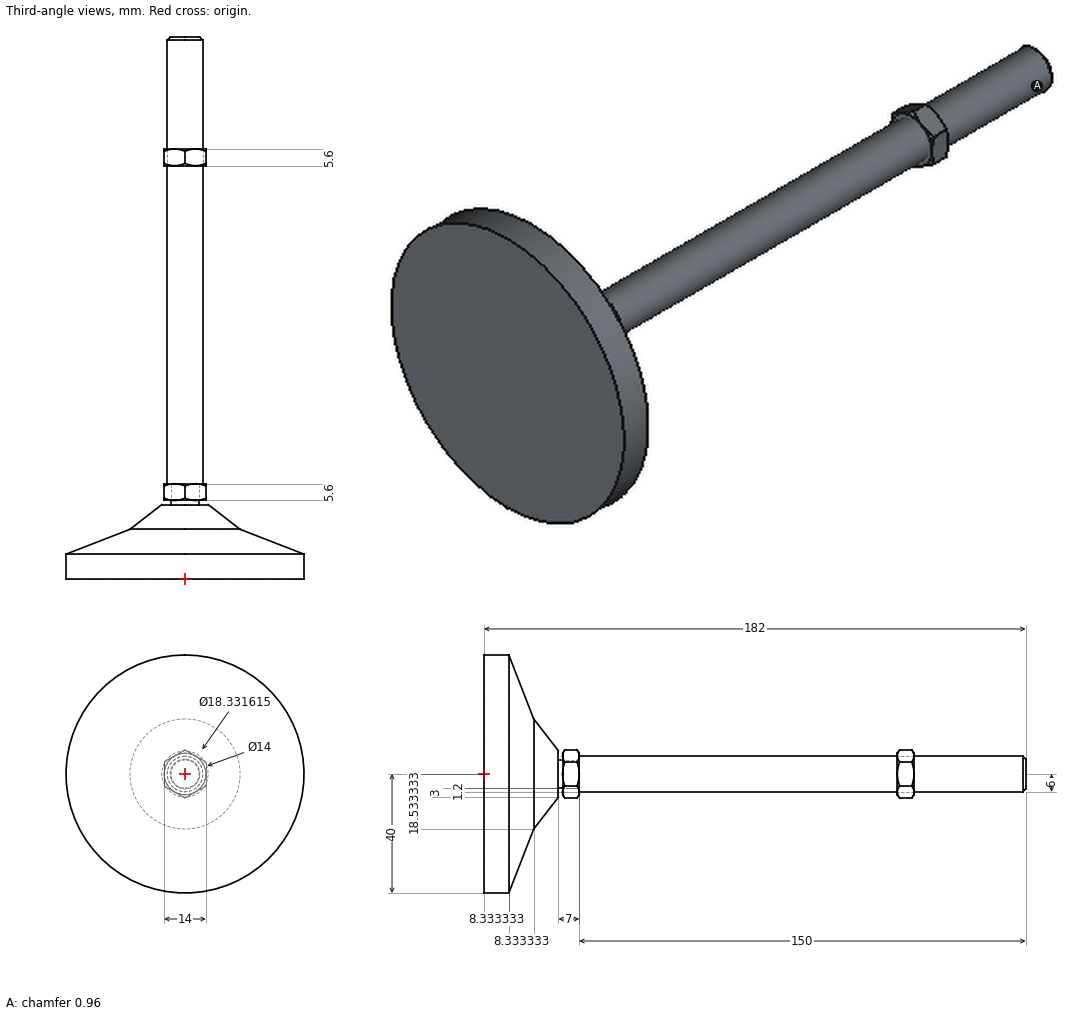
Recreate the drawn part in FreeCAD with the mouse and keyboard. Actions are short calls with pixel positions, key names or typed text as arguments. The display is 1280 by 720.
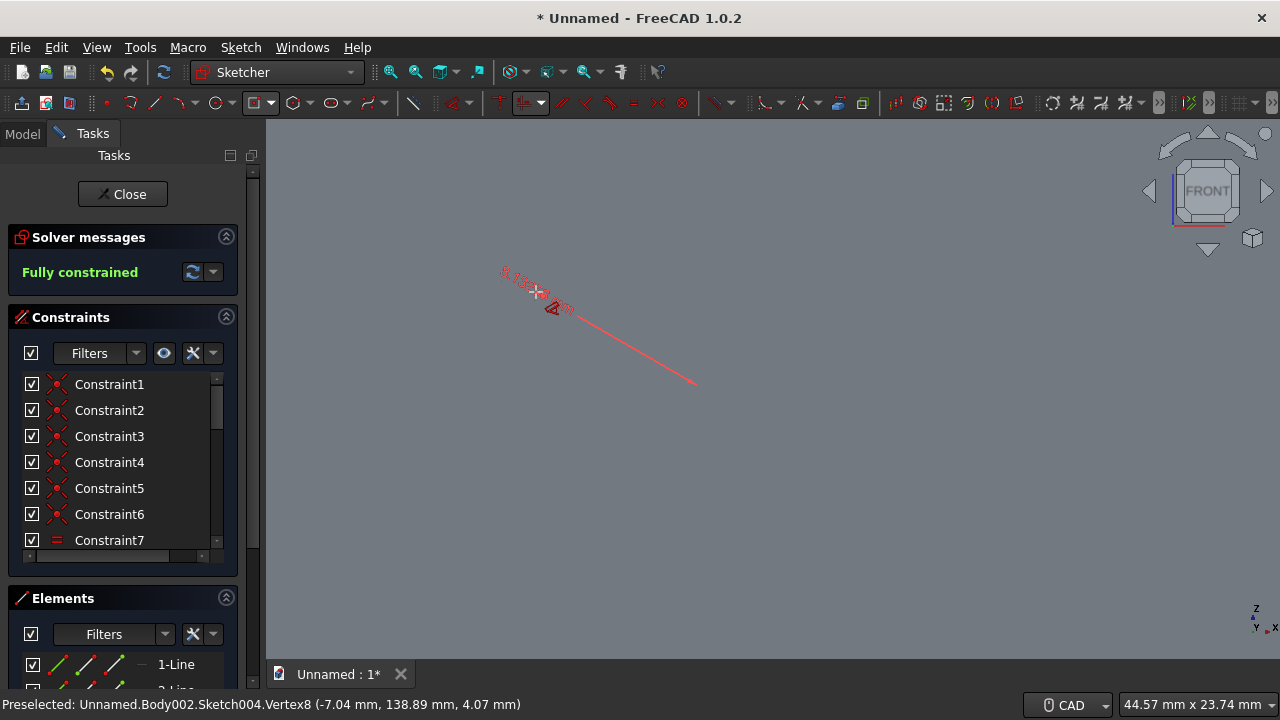
click(857, 477)
click(623, 511)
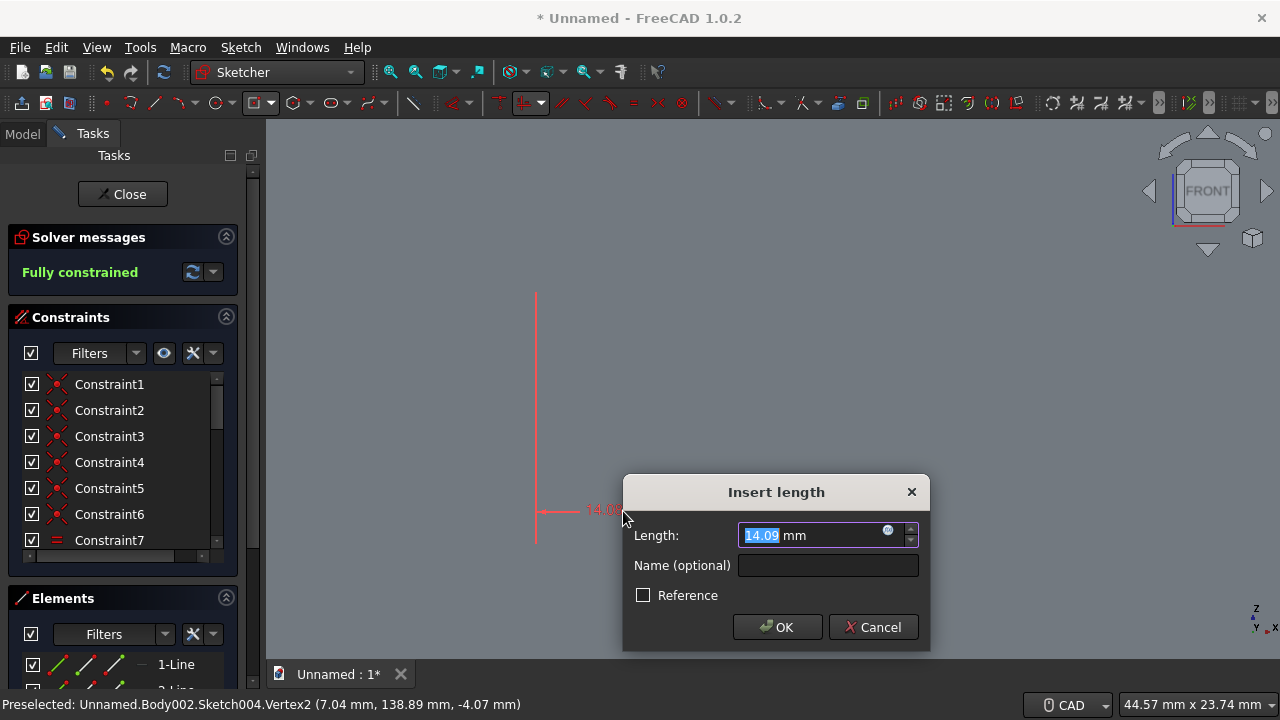
text(14)
key(Return)
key(Escape)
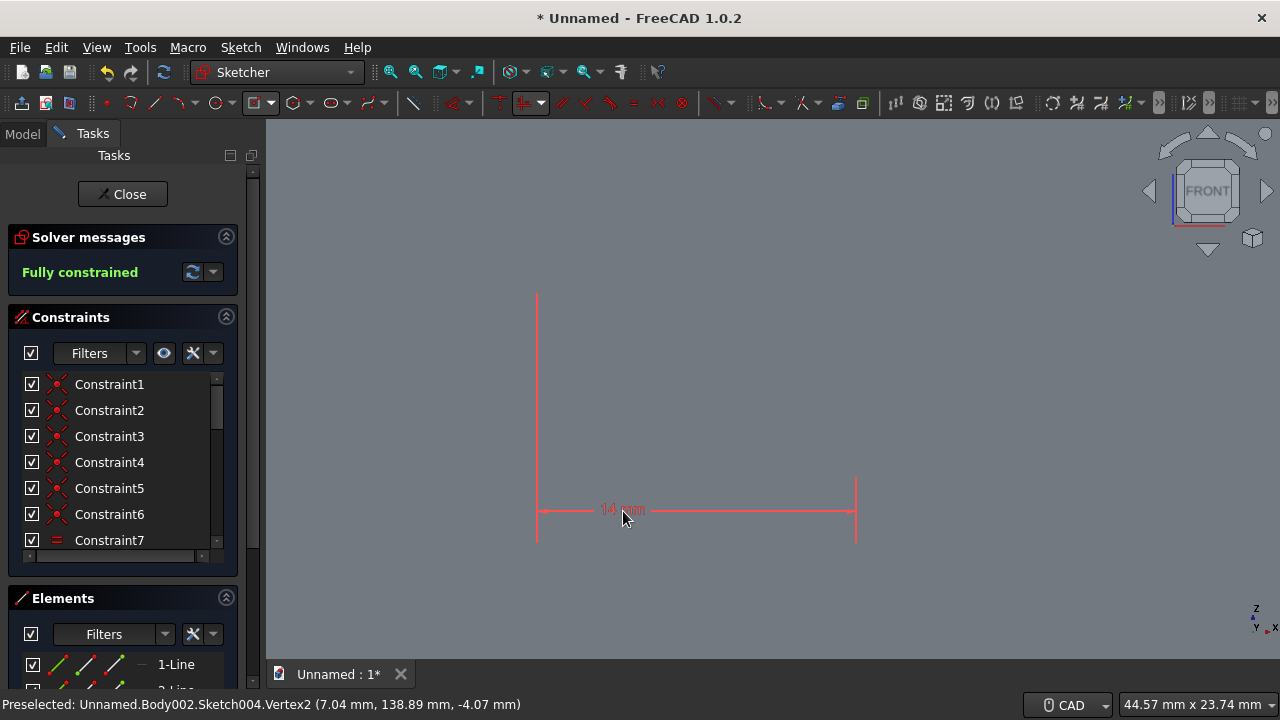
click(123, 194)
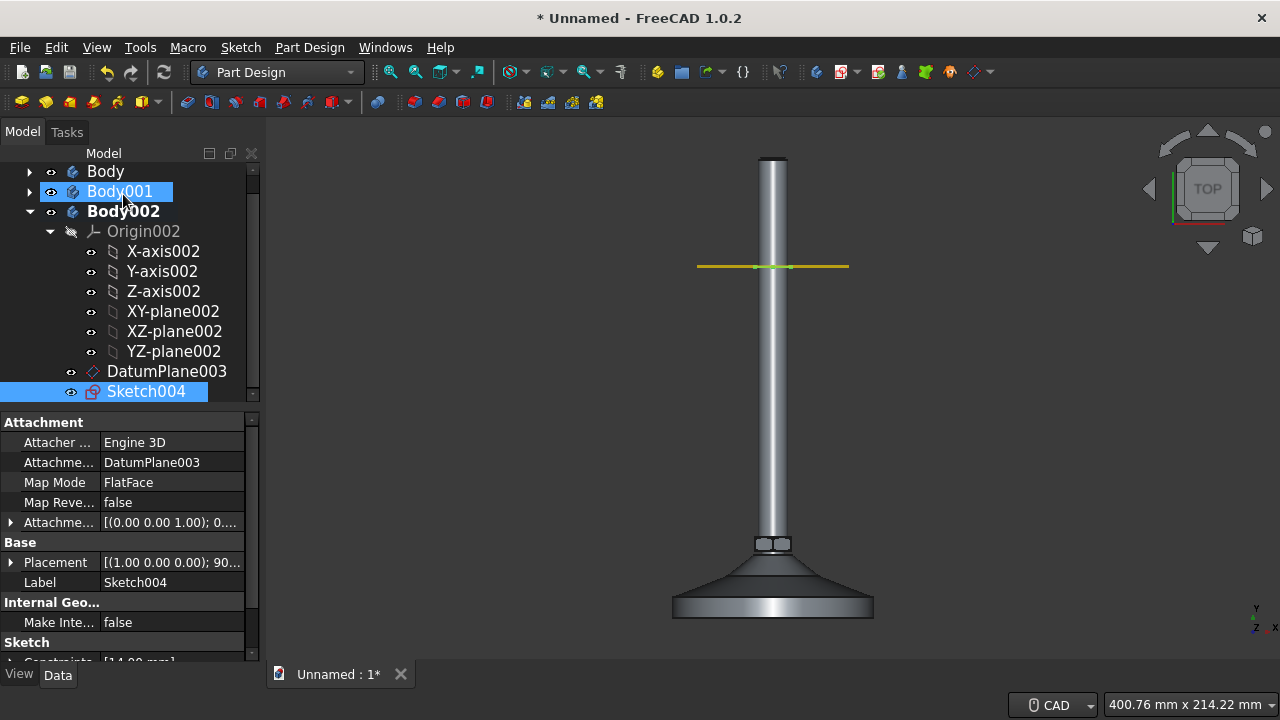
click(22, 102)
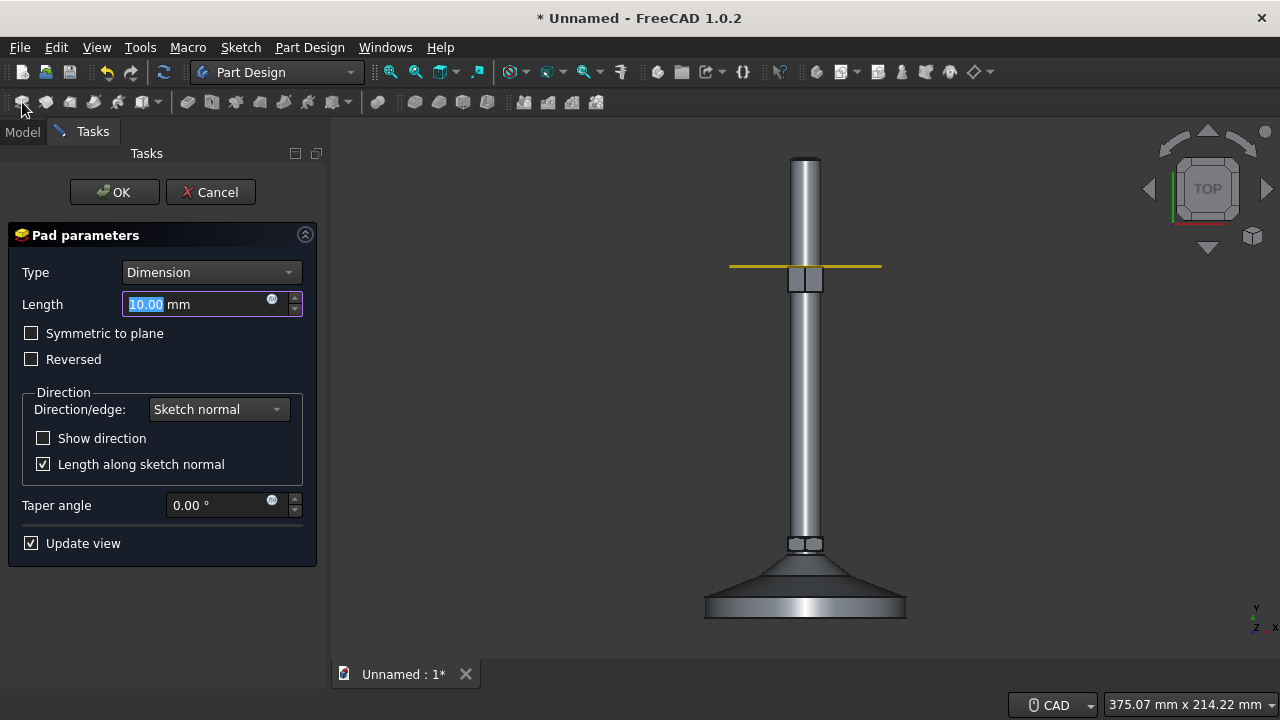
text(5.6)
key(Tab)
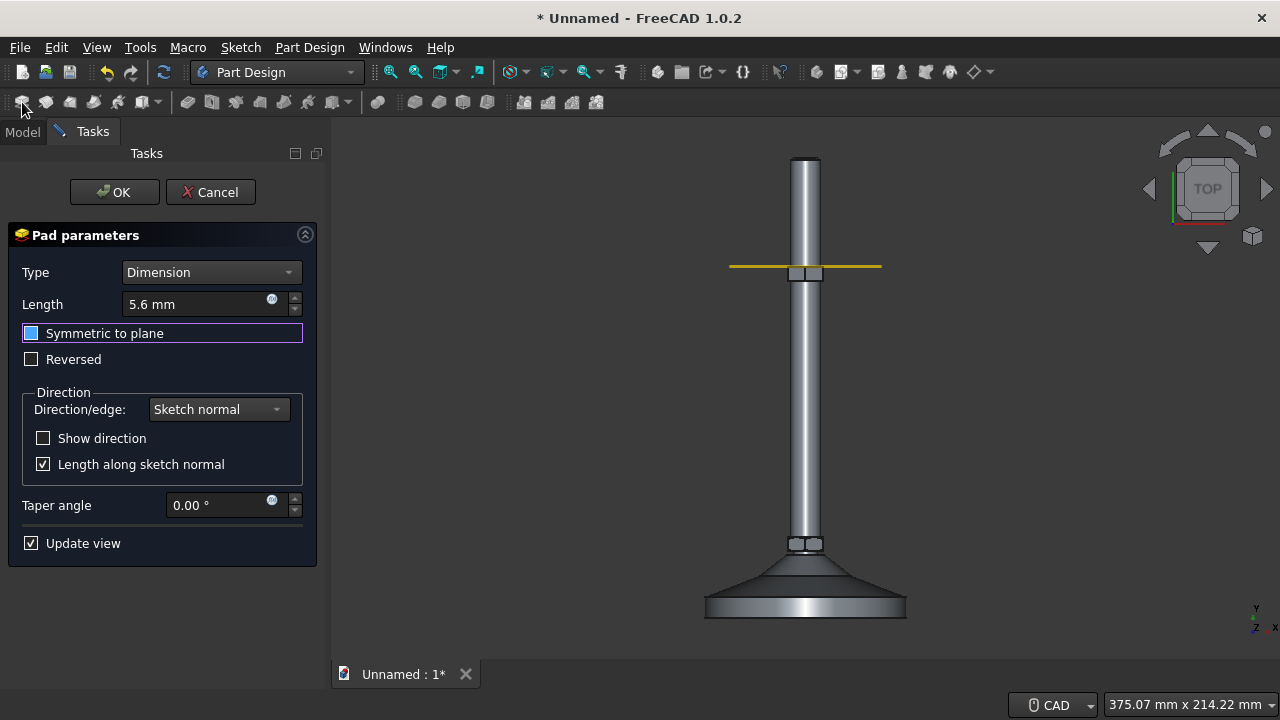
click(30, 359)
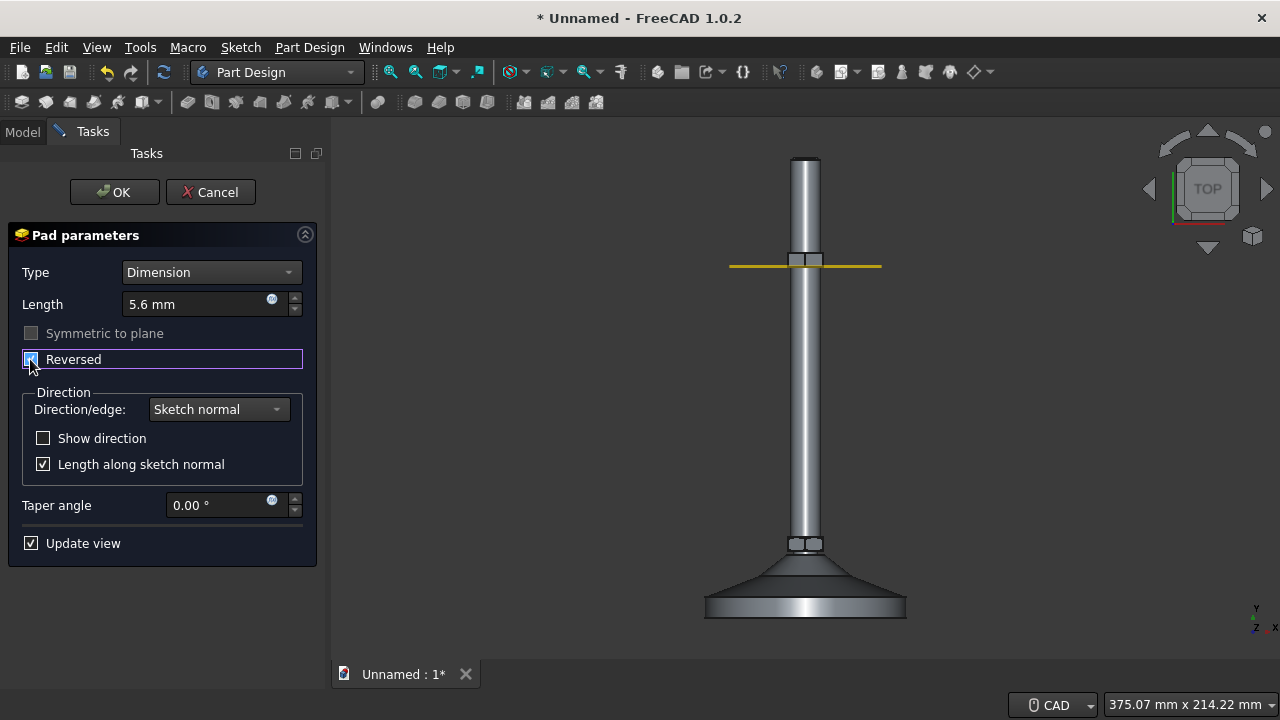
click(115, 192)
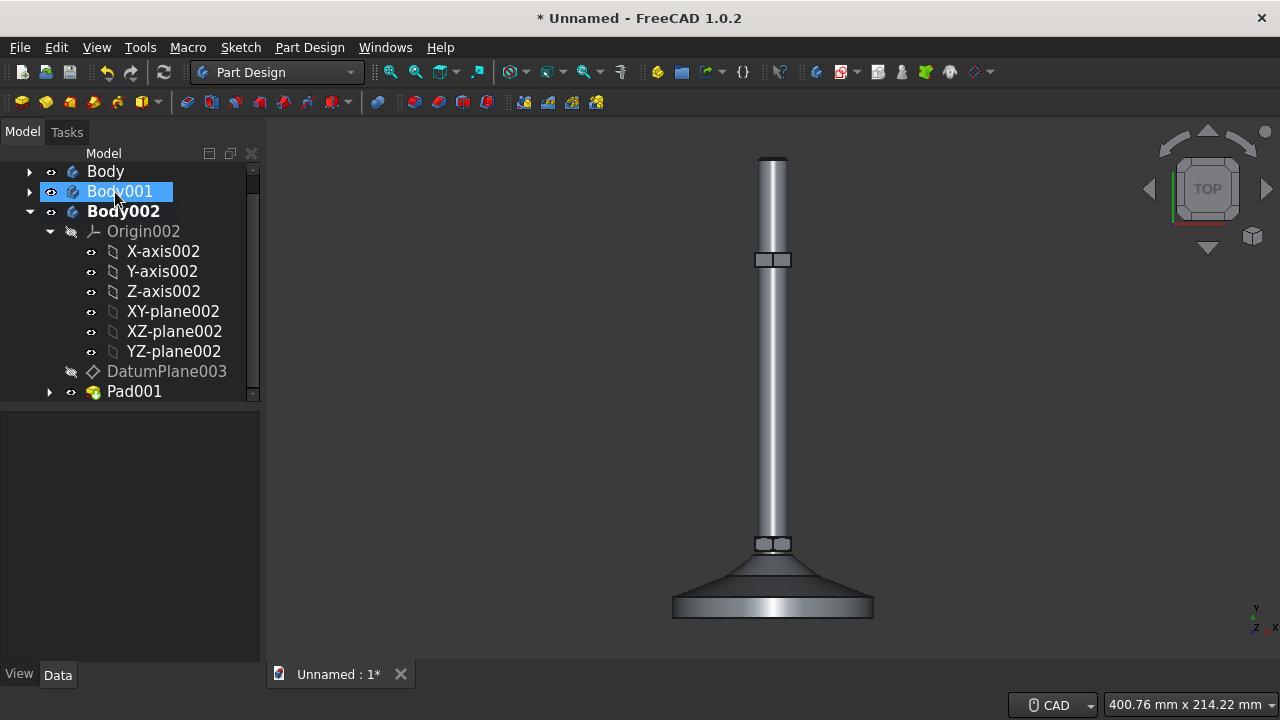
click(392, 72)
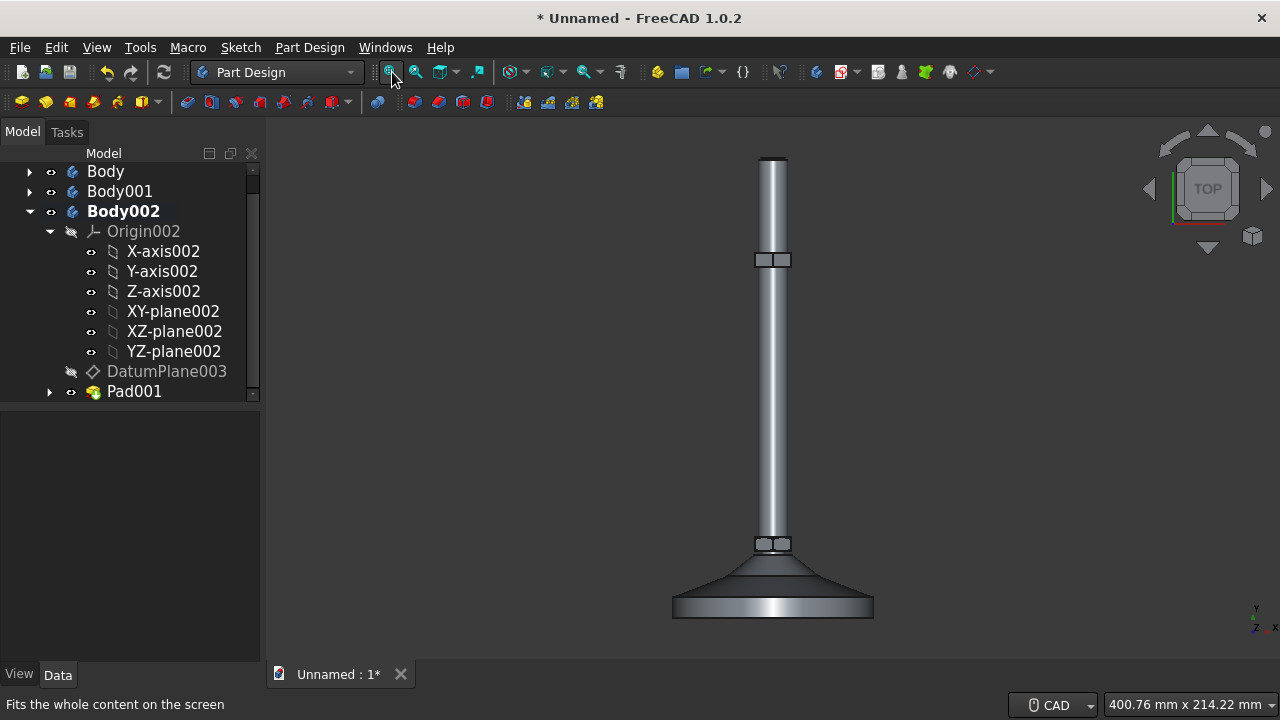
key(4)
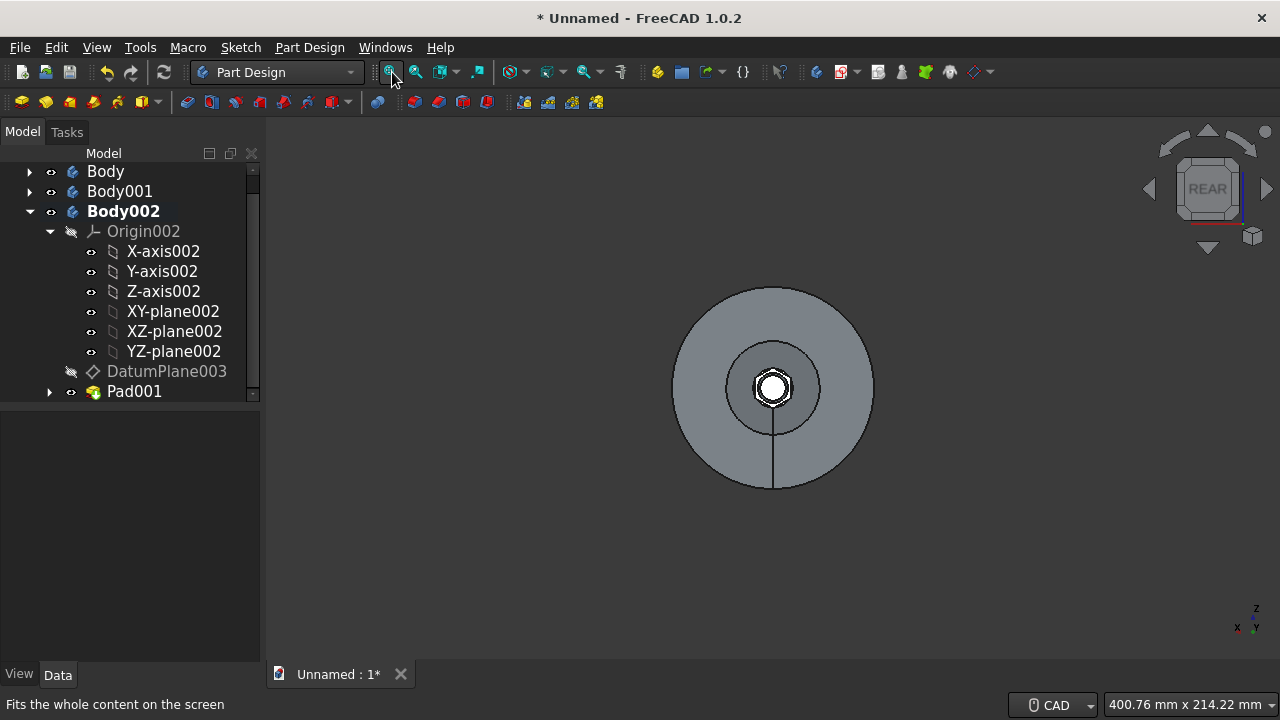
click(392, 72)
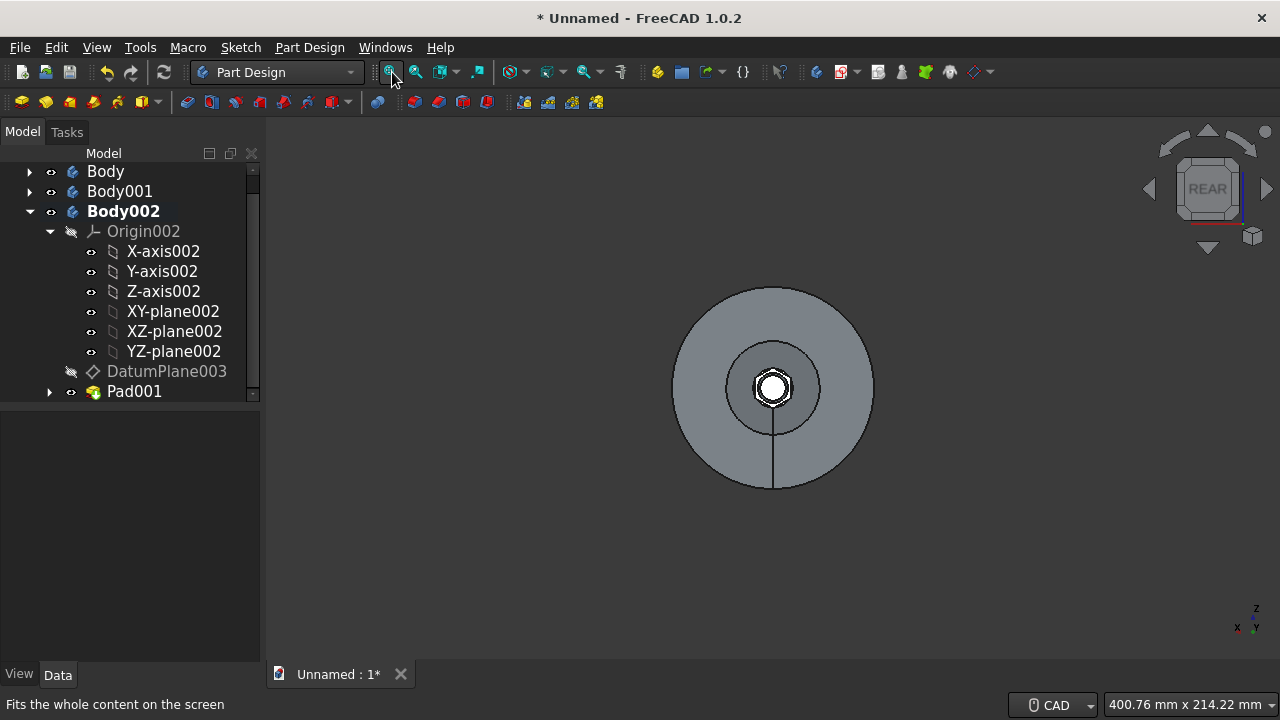
key(5)